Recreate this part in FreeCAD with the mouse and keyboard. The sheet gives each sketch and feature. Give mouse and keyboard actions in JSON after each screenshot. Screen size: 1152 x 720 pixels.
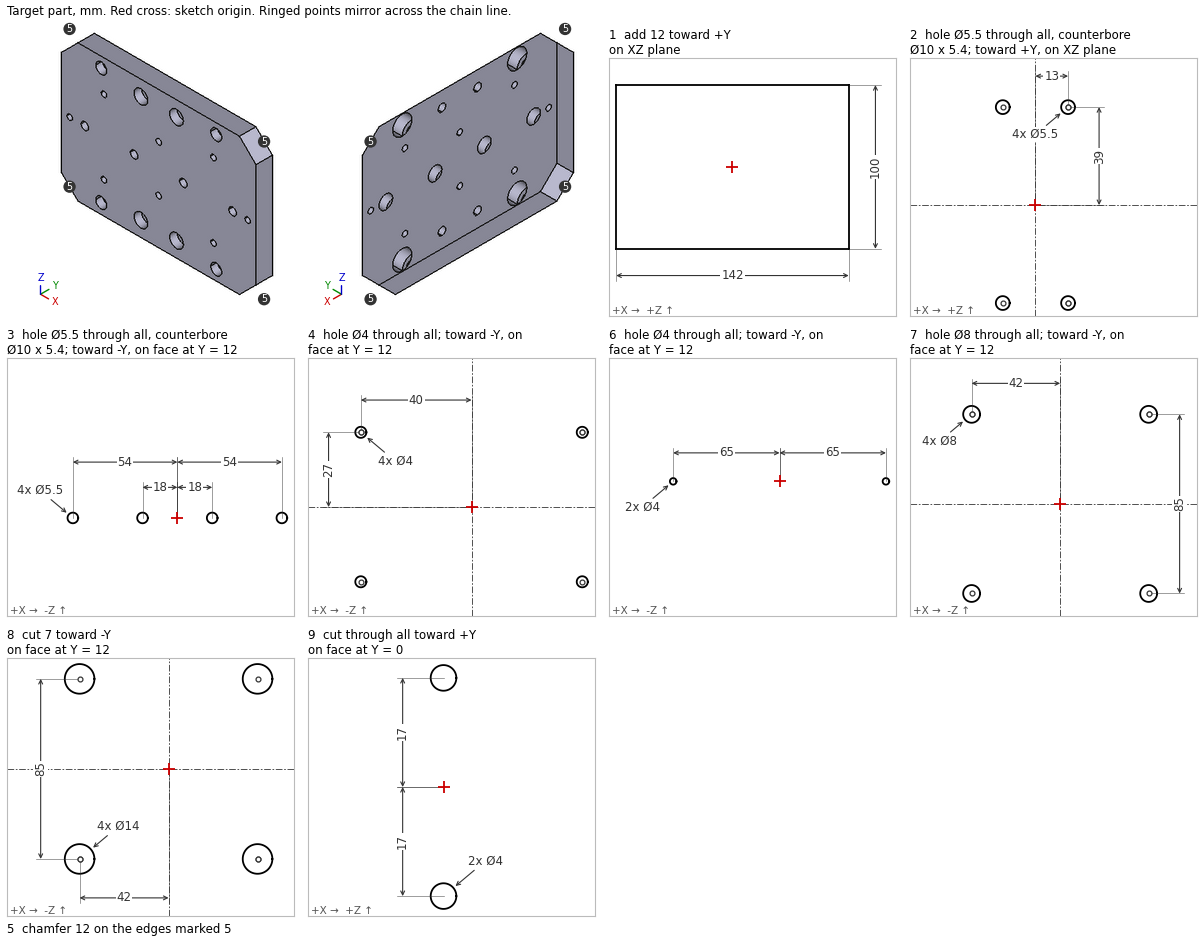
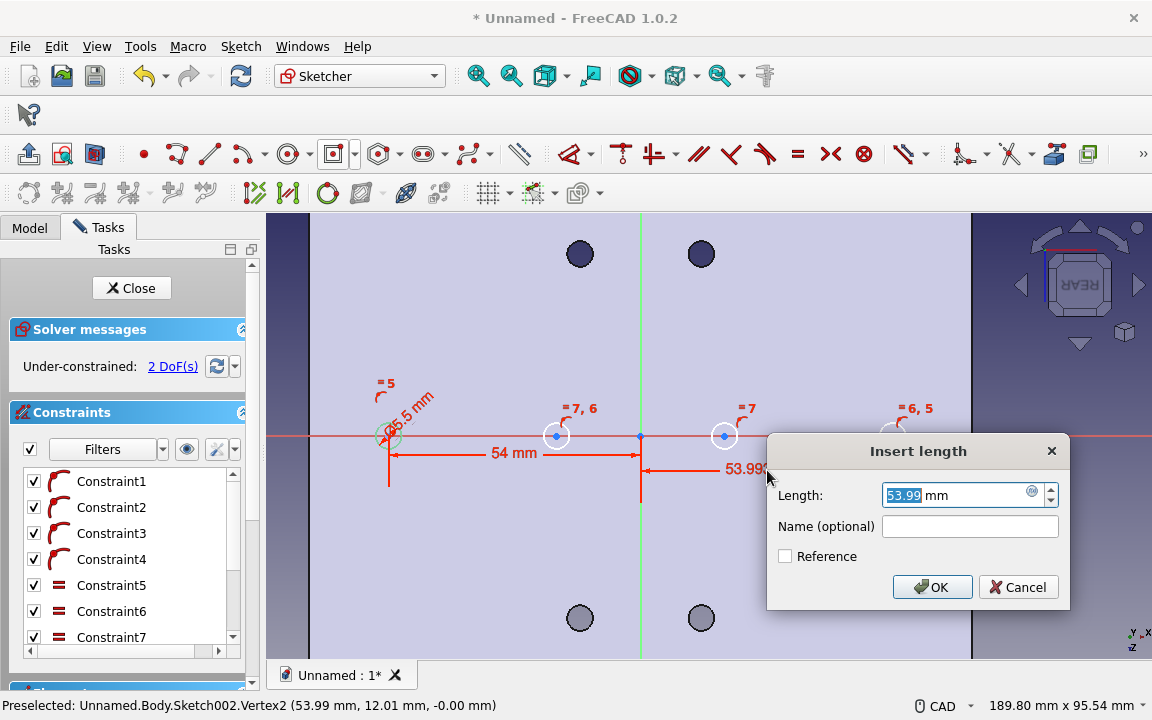
{"action": "type", "text": "54"}
{"action": "key", "text": "Return"}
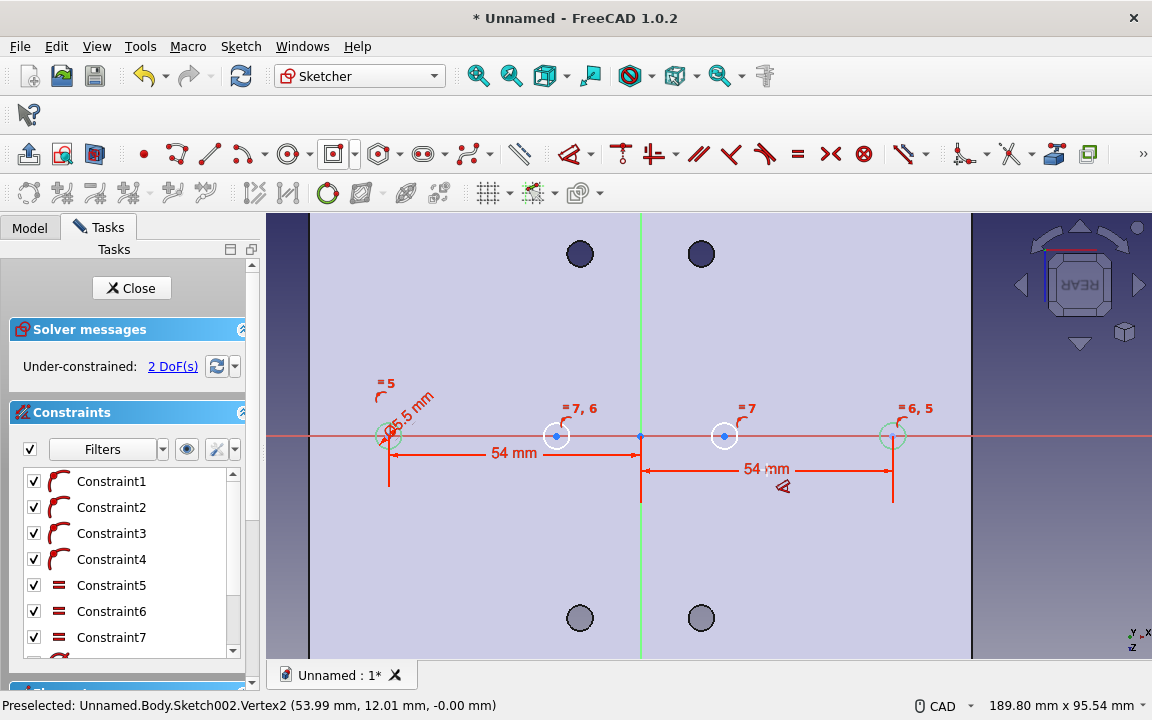
{"action": "left_click", "coordinate": [557, 436]}
{"action": "left_click", "coordinate": [599, 470]}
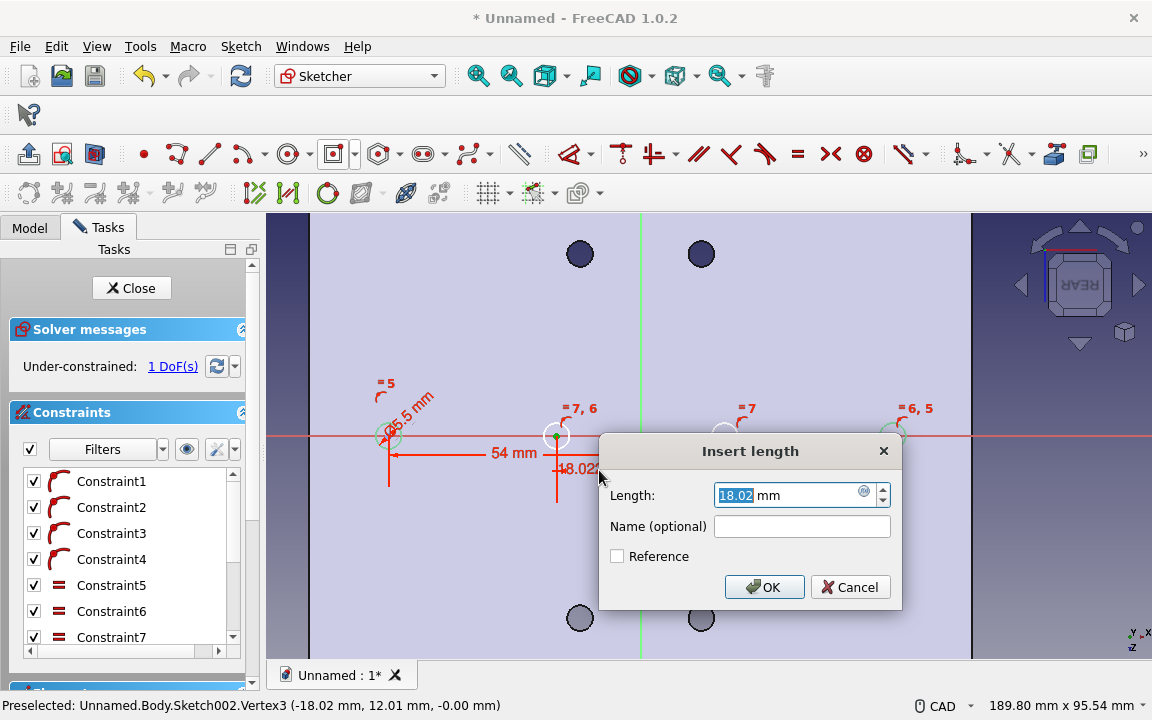
{"action": "type", "text": "18"}
{"action": "key", "text": "Return"}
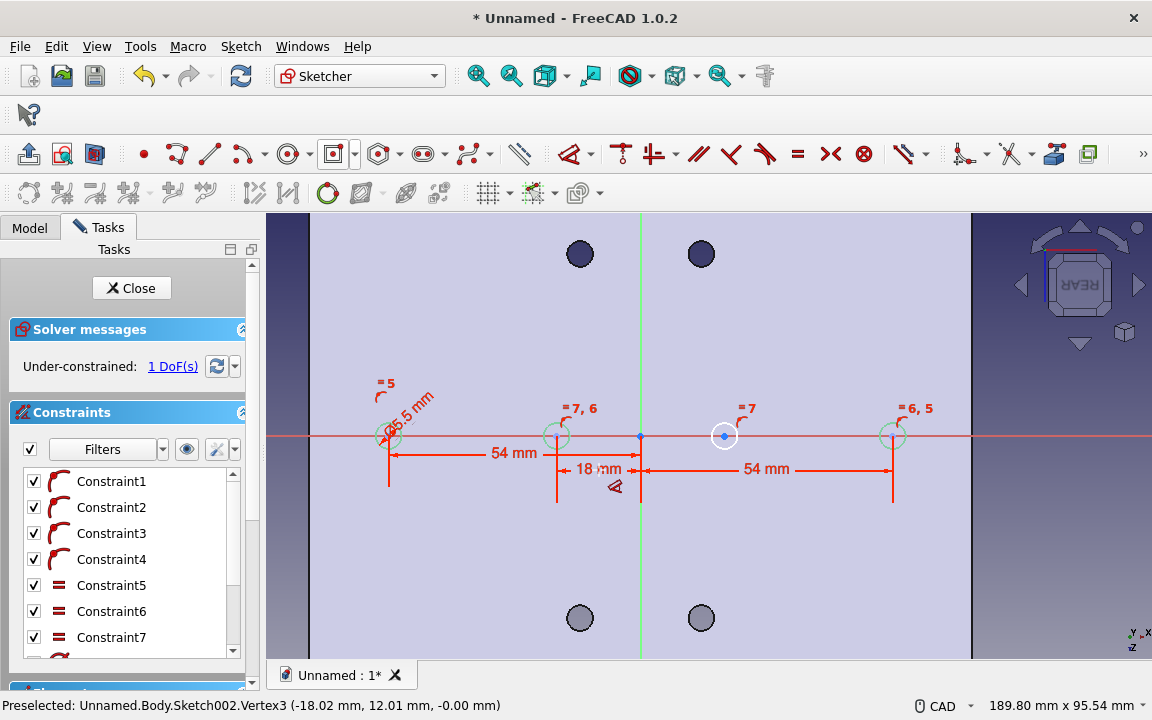
{"action": "left_click", "coordinate": [725, 436]}
{"action": "left_click", "coordinate": [683, 470]}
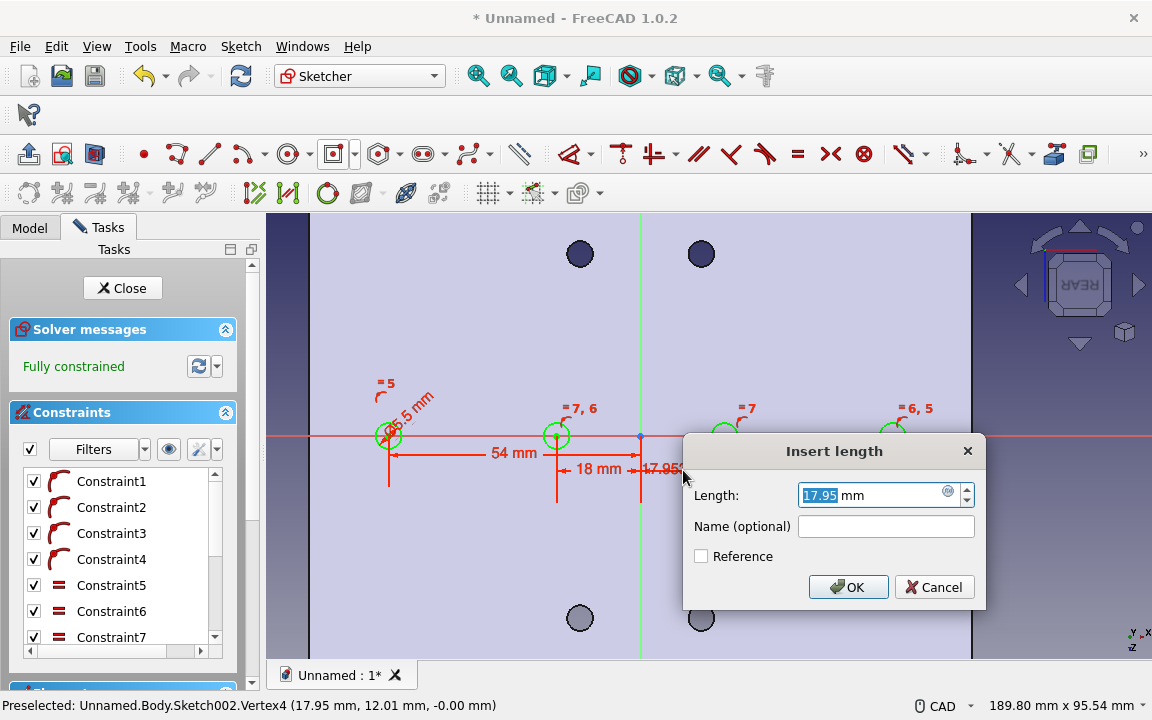
{"action": "type", "text": "18"}
{"action": "key", "text": "Return"}
{"action": "key", "text": "Escape"}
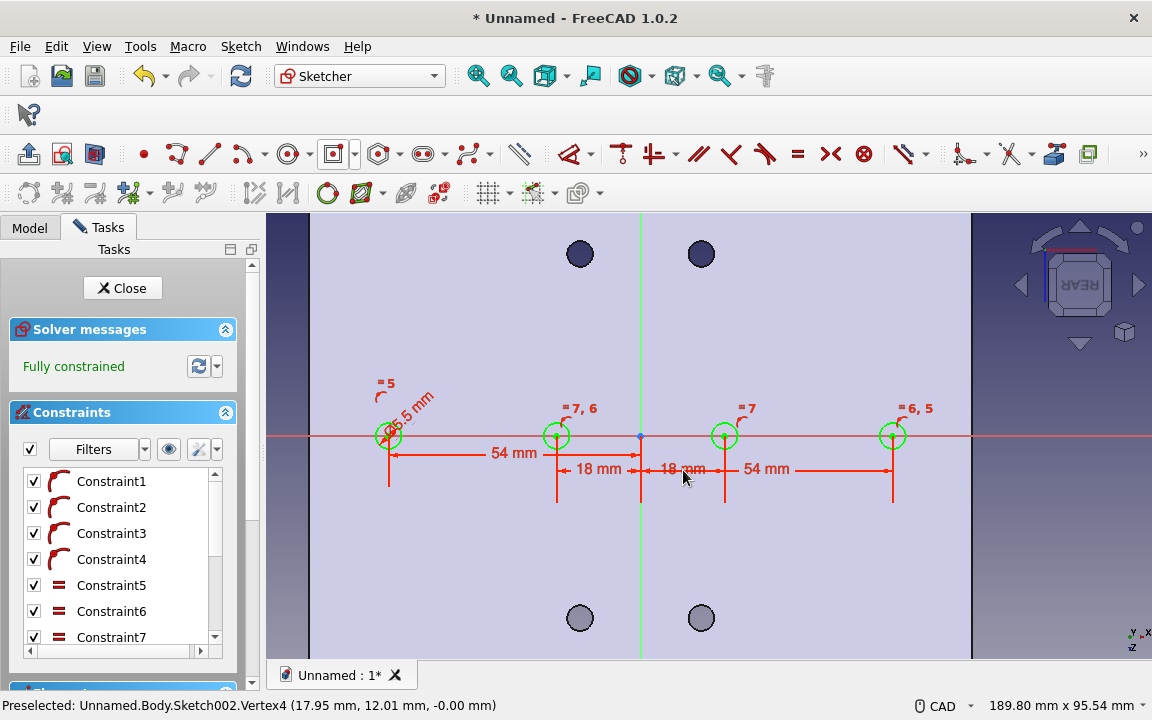
{"action": "left_click", "coordinate": [123, 288]}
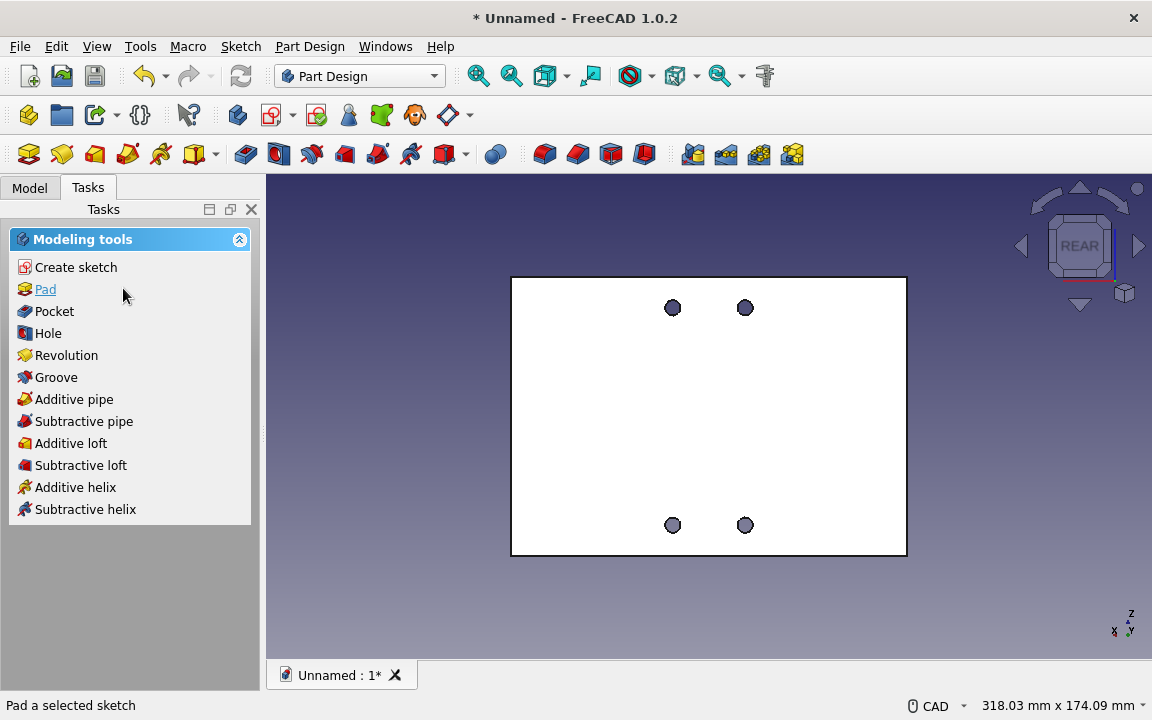
{"action": "left_click", "coordinate": [279, 154]}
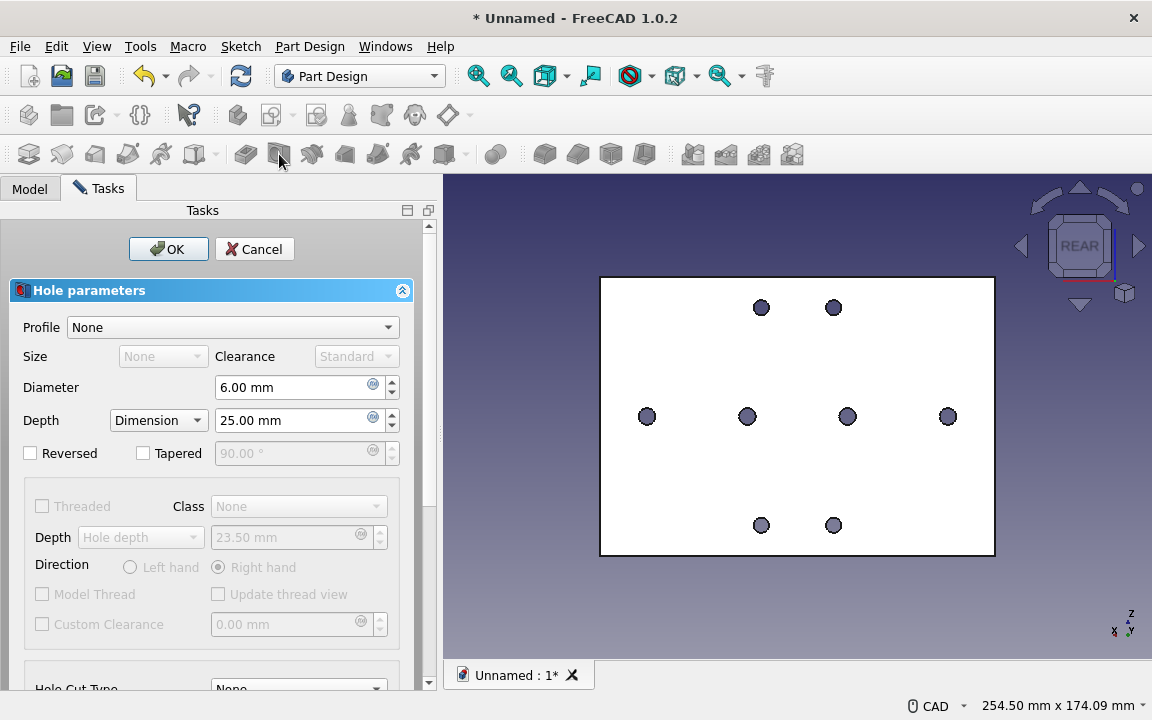
{"action": "triple_click", "coordinate": [300, 388]}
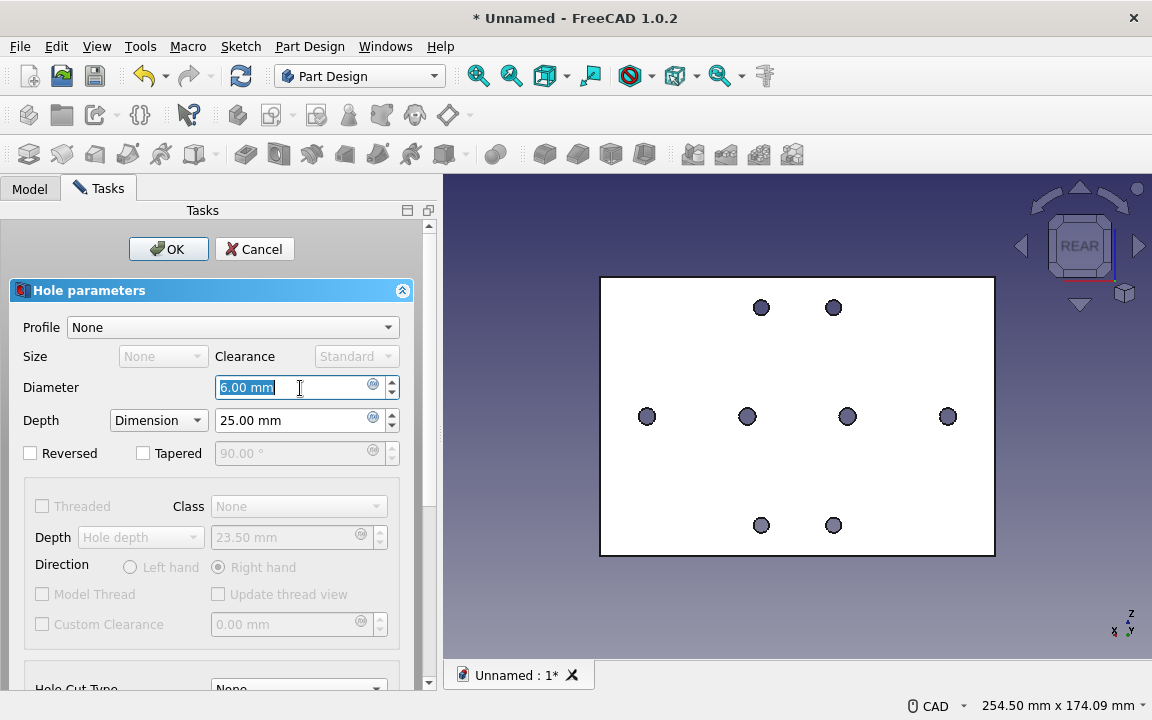
{"action": "type", "text": "5.5"}
{"action": "key", "text": "Tab"}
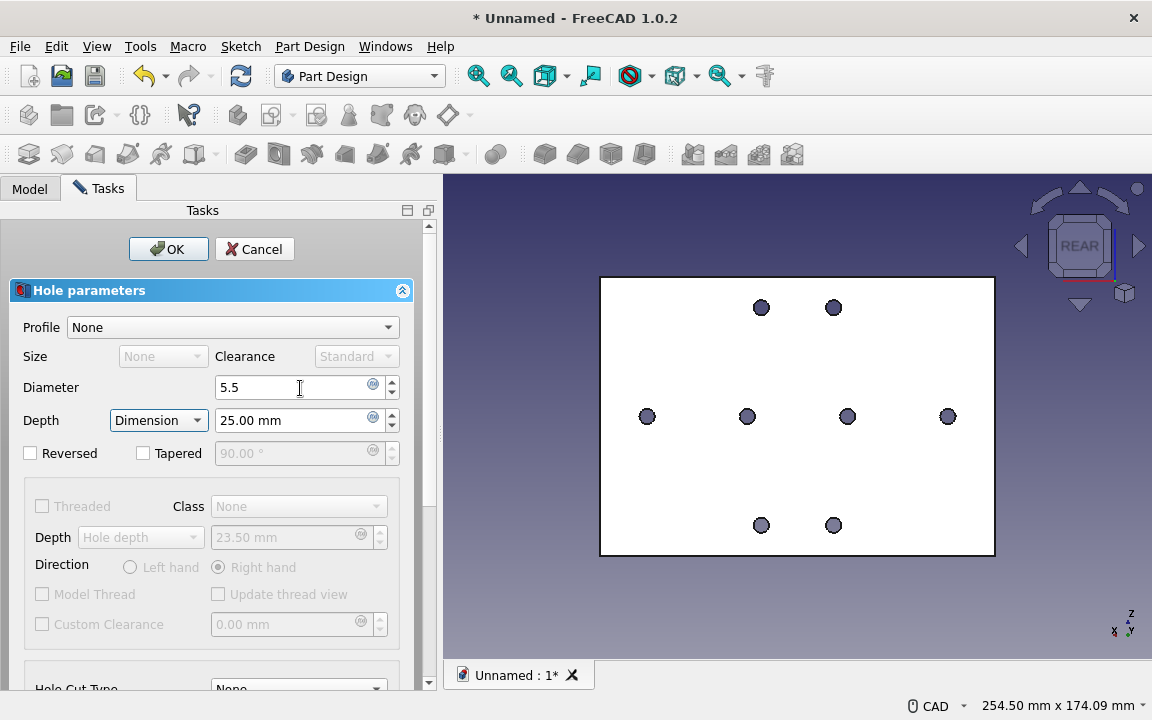
{"action": "left_click", "coordinate": [160, 420]}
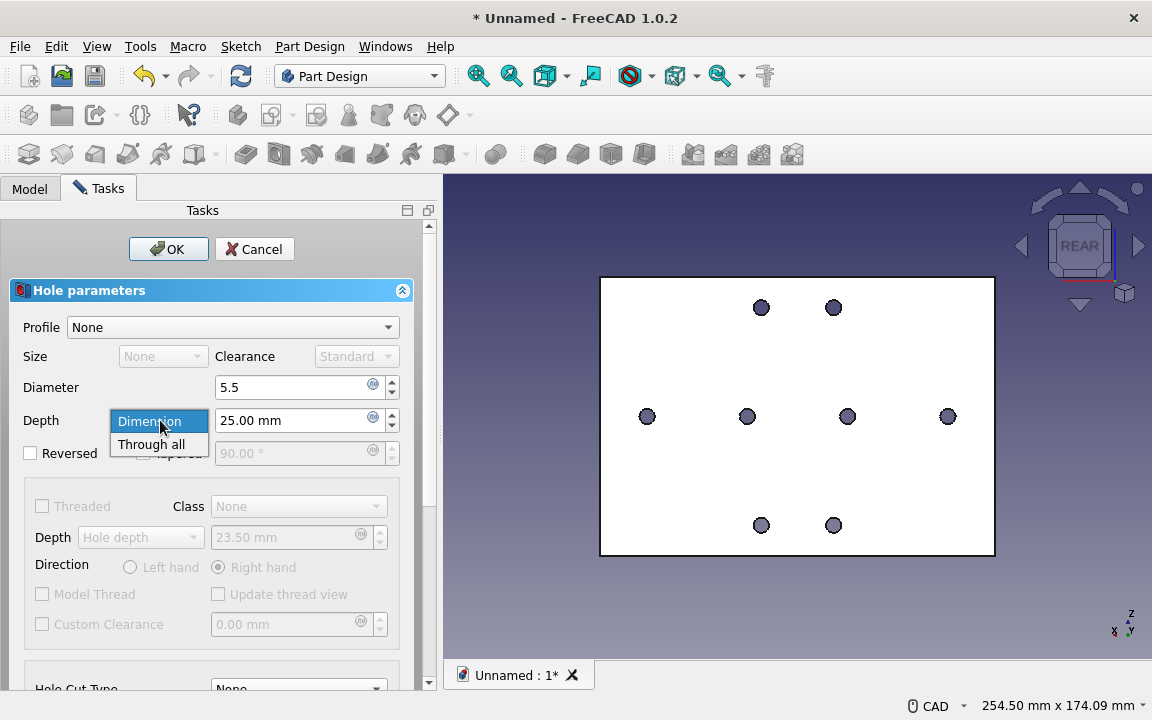
{"action": "left_click", "coordinate": [158, 444]}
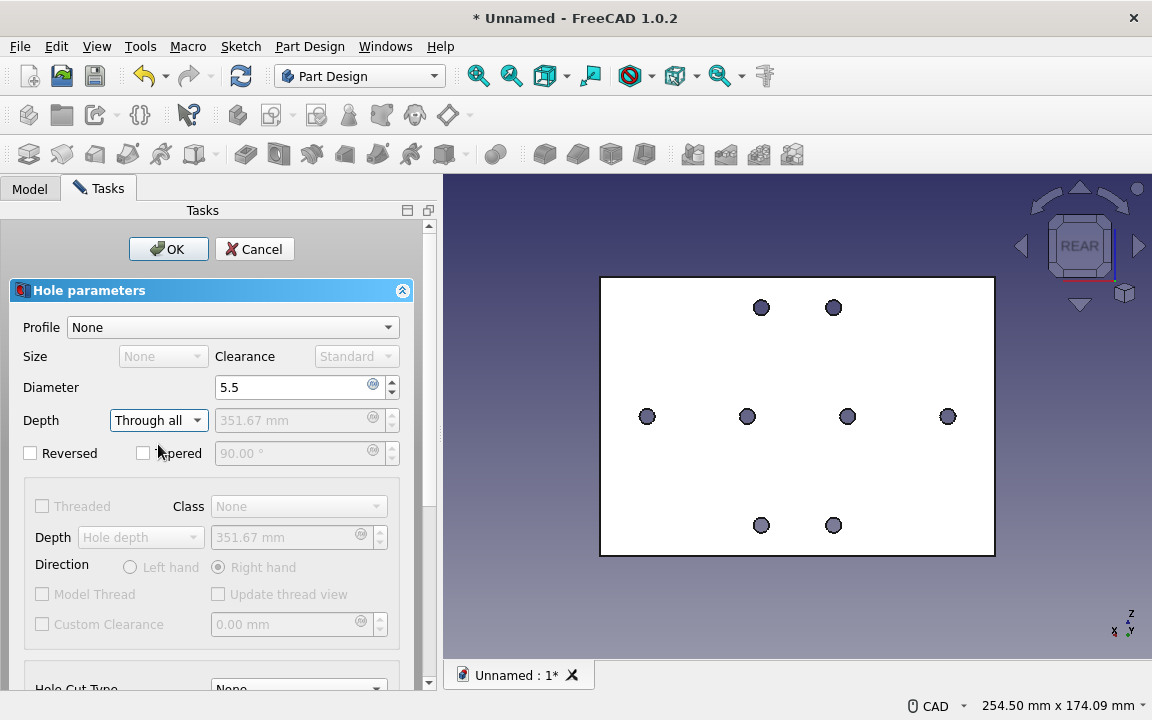
{"action": "scroll", "coordinate": [429, 455], "scroll_direction": "down", "scroll_amount": 2}